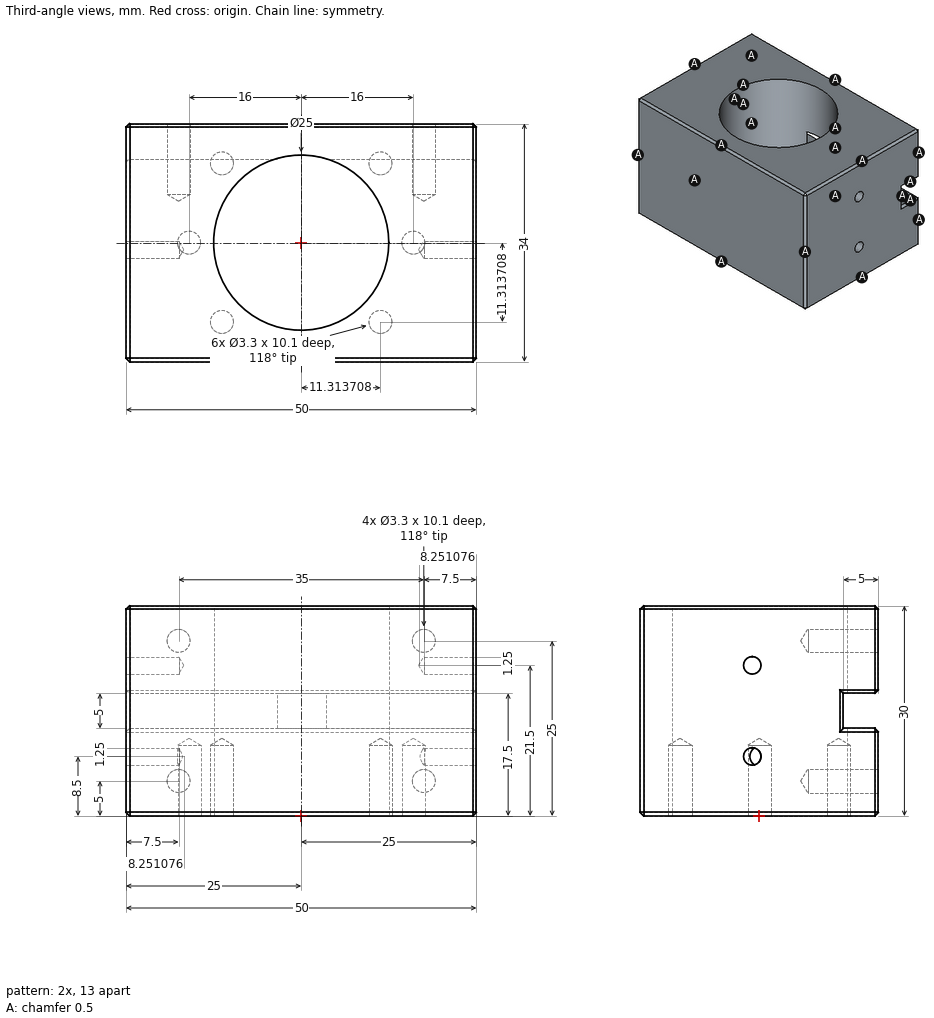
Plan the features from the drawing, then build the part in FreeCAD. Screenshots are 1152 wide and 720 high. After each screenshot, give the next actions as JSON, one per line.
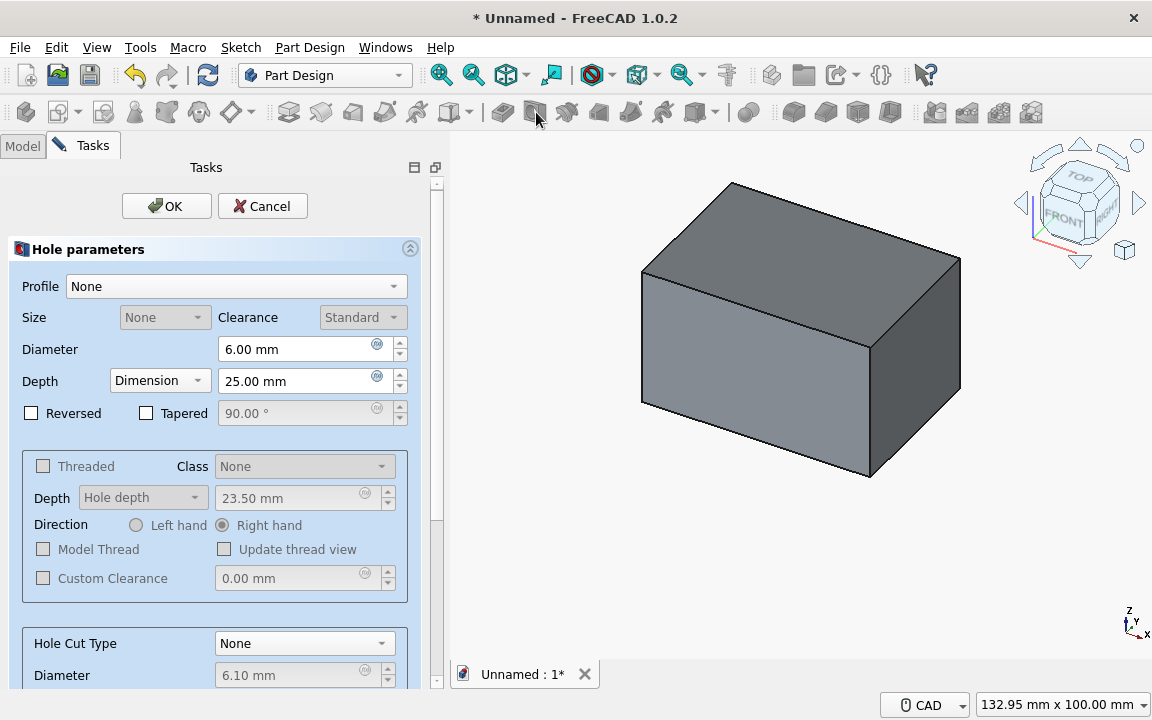
{"action": "triple_click", "coordinate": [305, 349]}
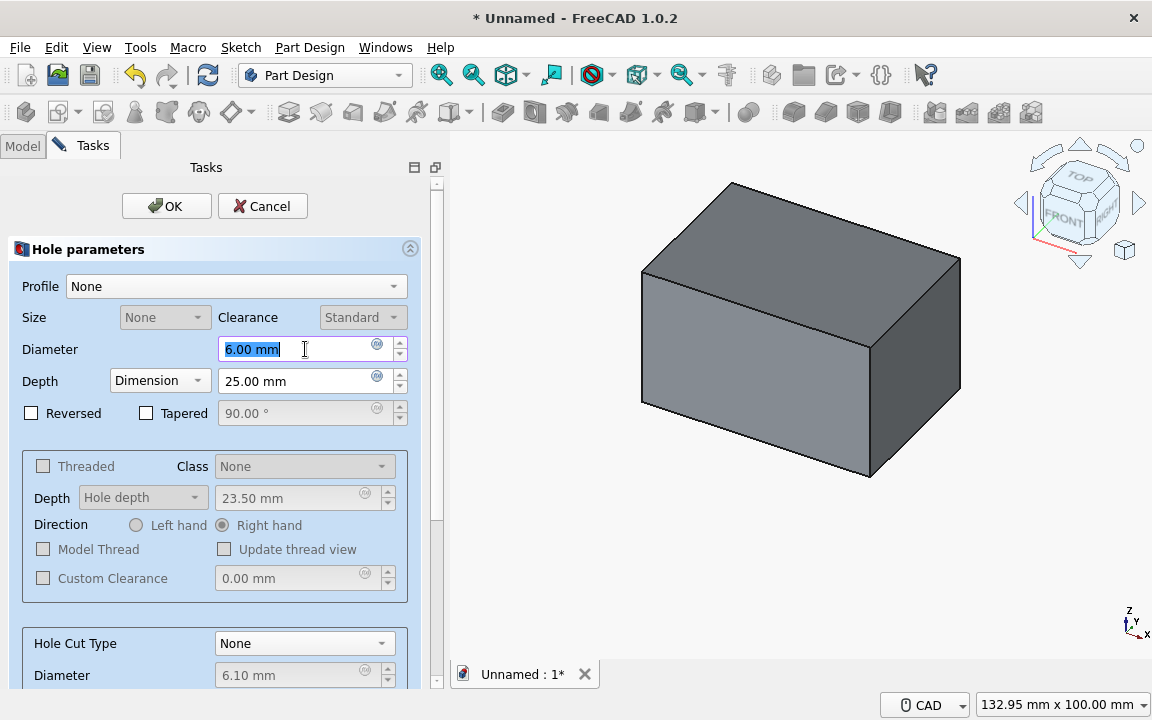
{"action": "type", "text": "3.3"}
{"action": "key", "text": "Tab"}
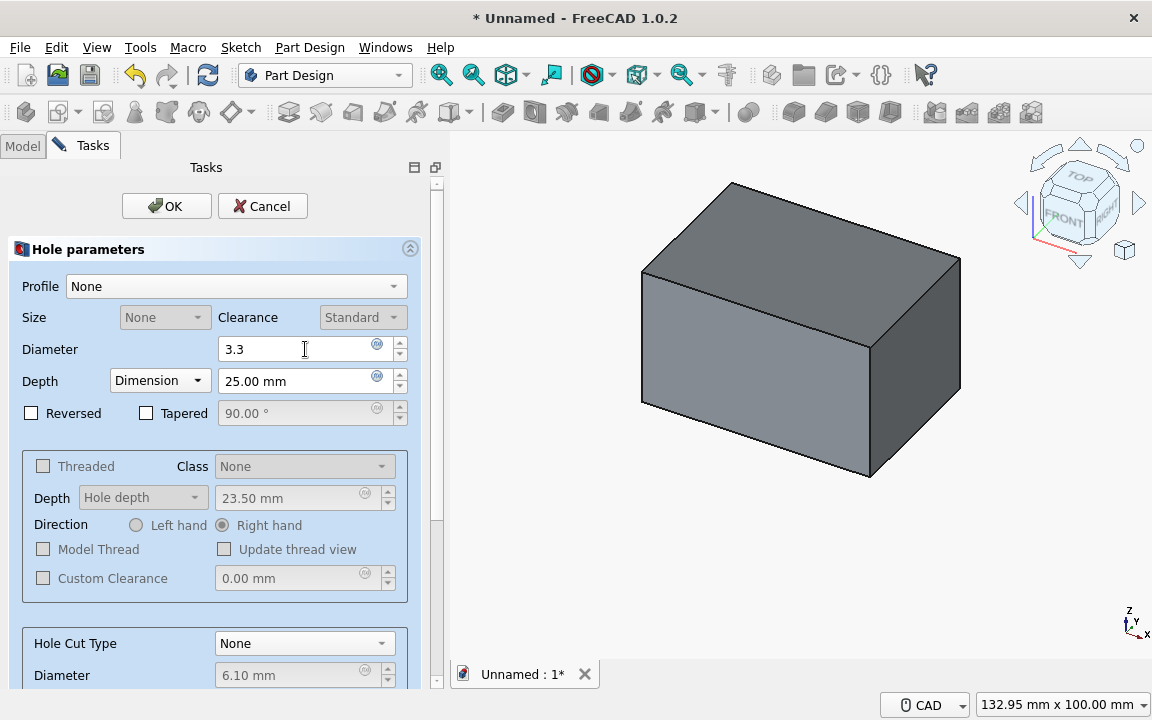
{"action": "triple_click", "coordinate": [305, 381]}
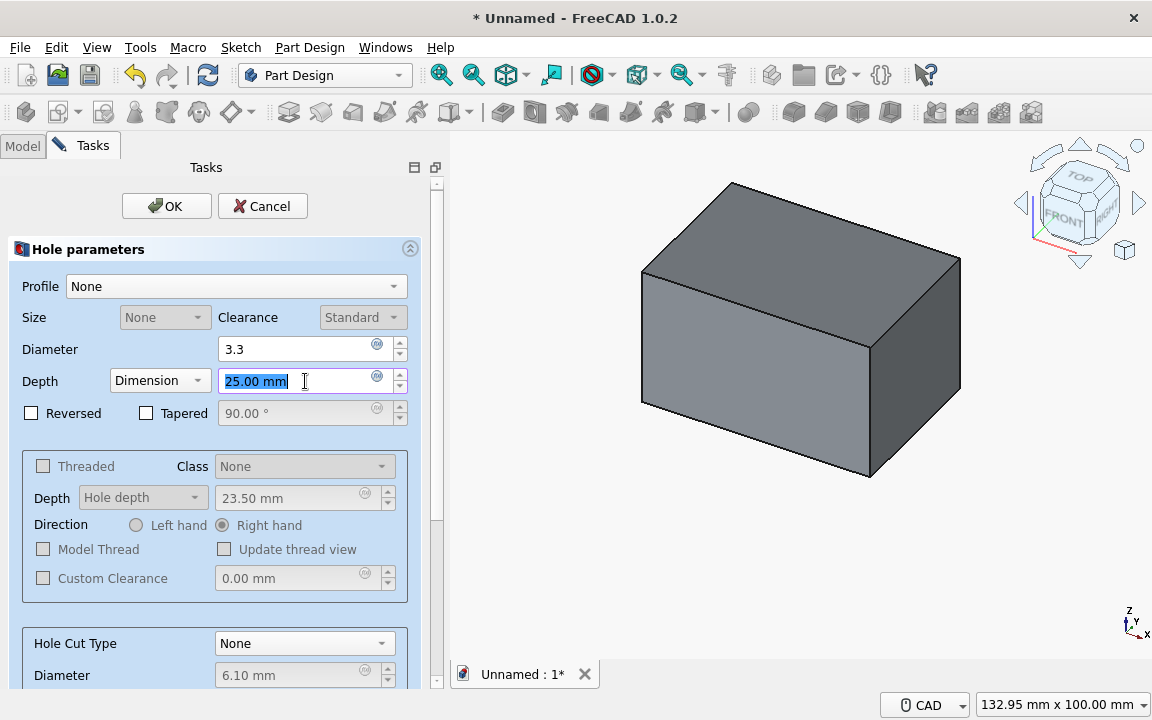
{"action": "type", "text": "10.1"}
{"action": "key", "text": "Tab"}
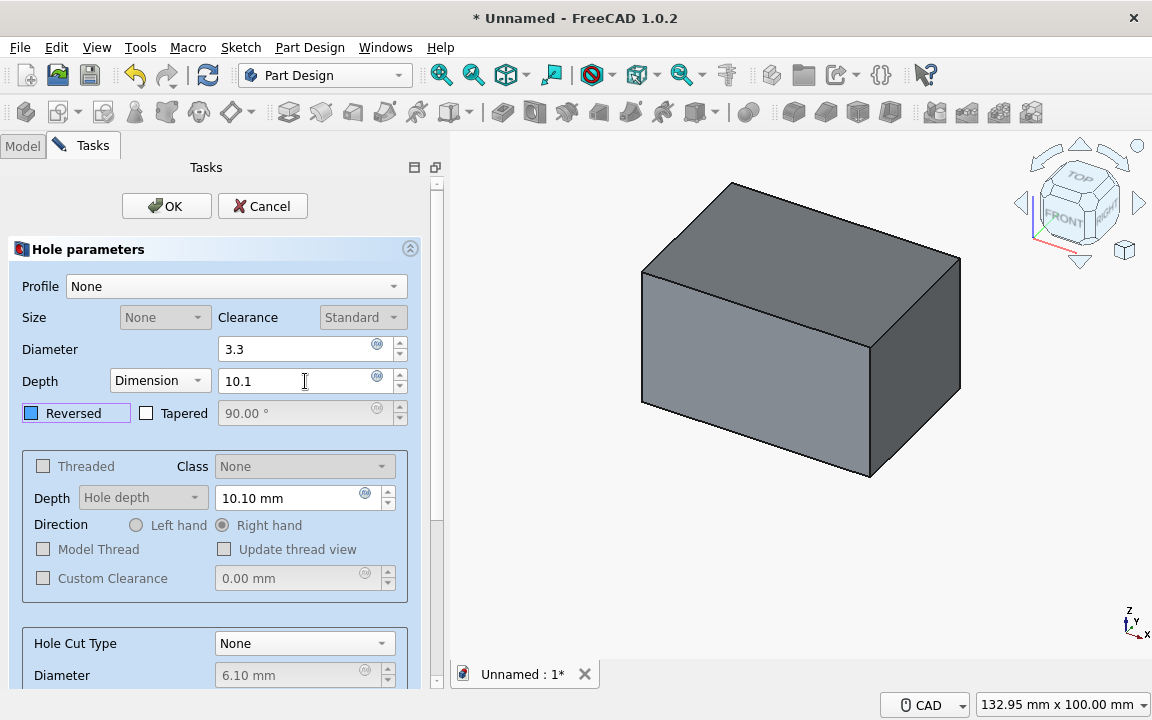
{"action": "left_click", "coordinate": [30, 413]}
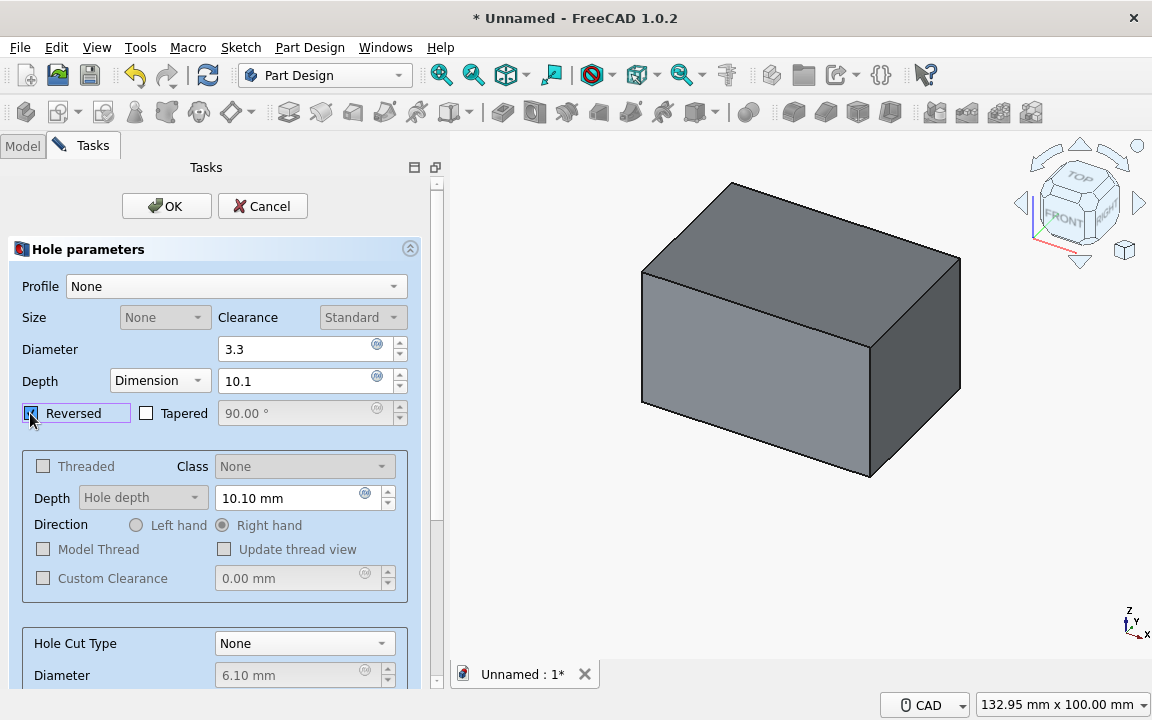
{"action": "left_click", "coordinate": [167, 206]}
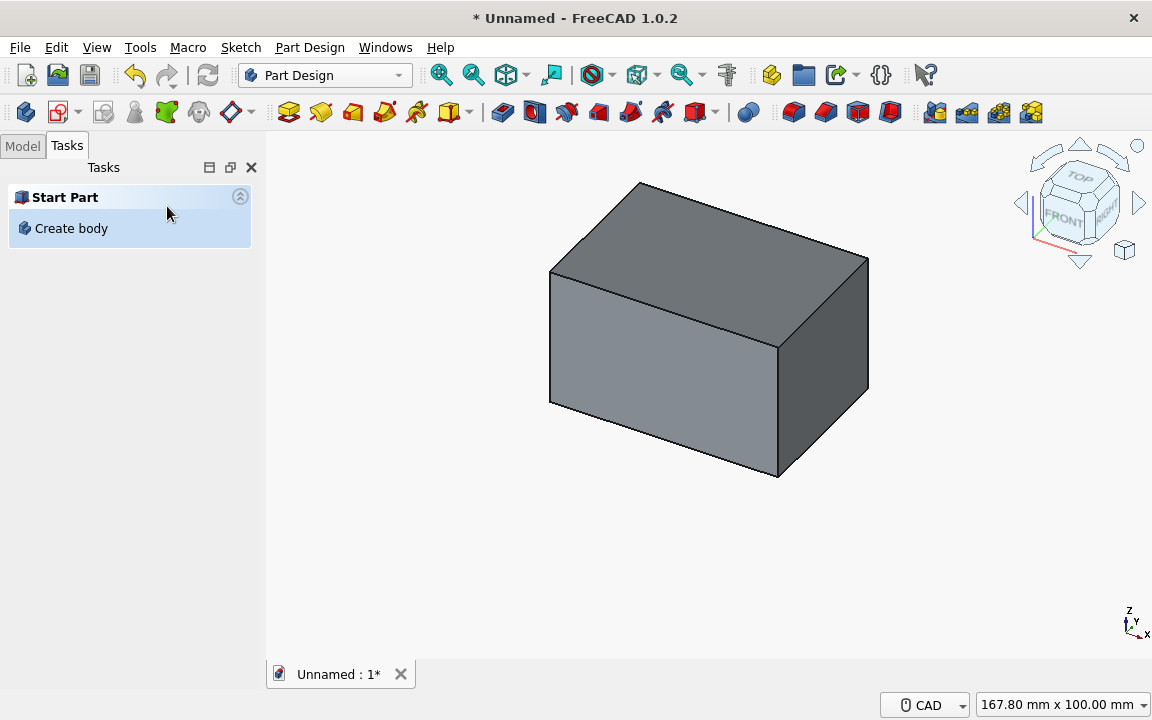
{"action": "left_click", "coordinate": [23, 145]}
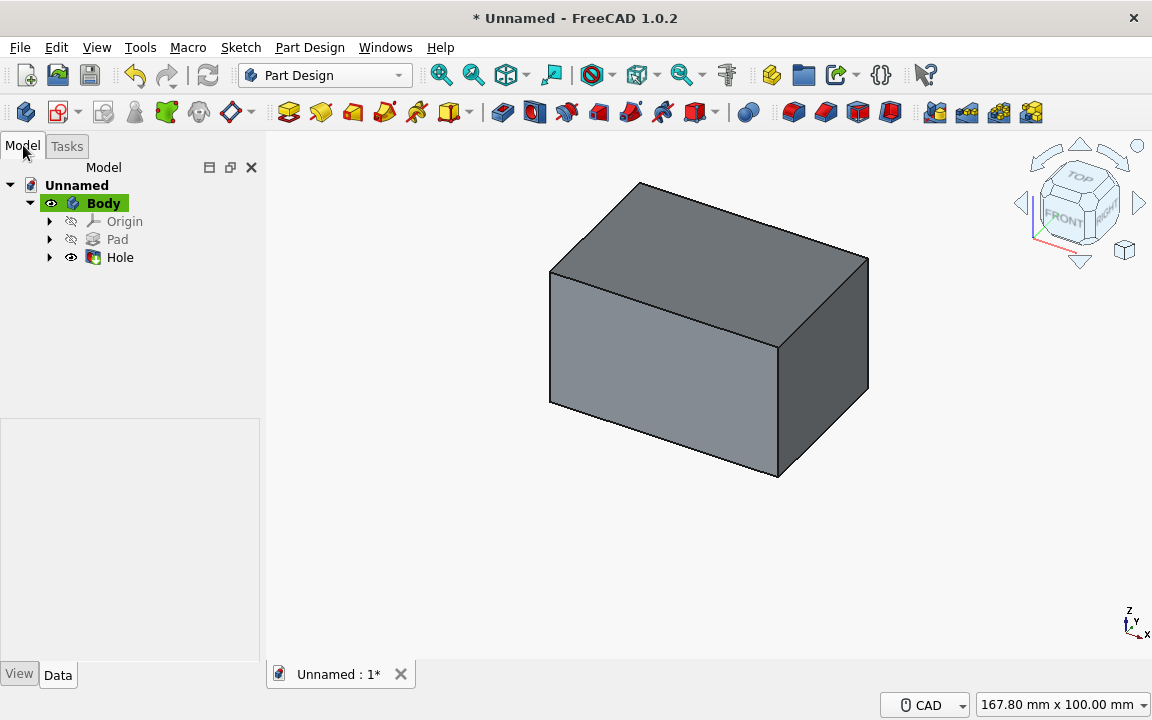
{"action": "left_click", "coordinate": [50, 221]}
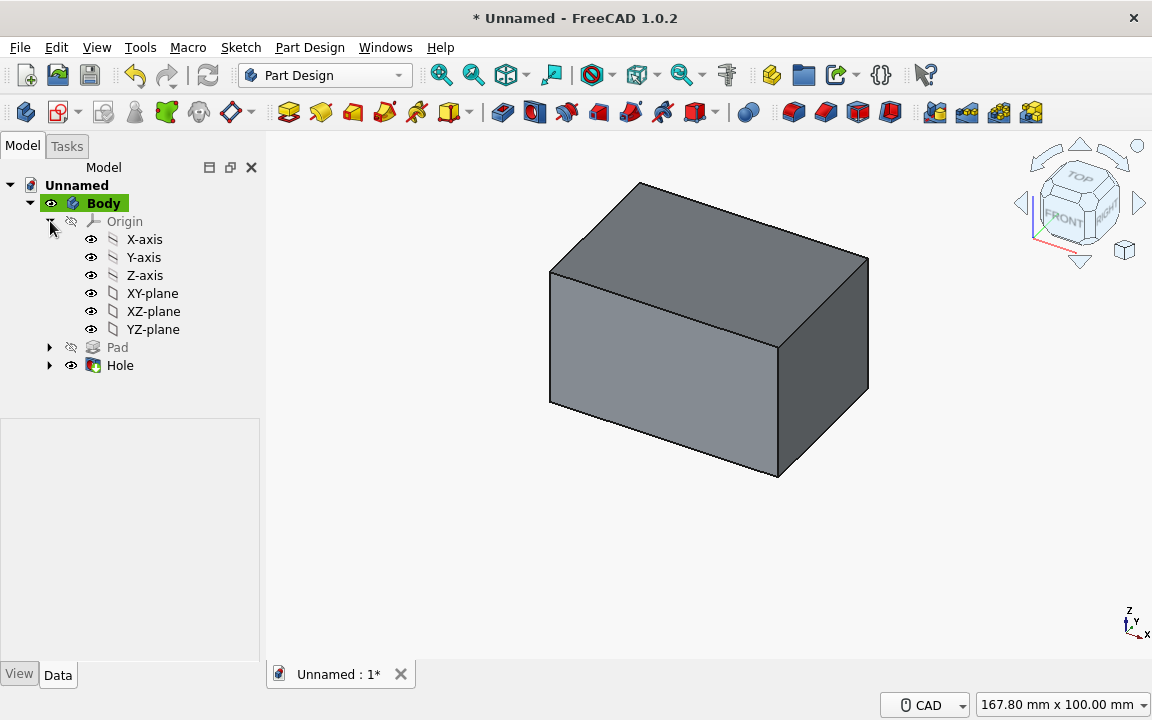
{"action": "left_click", "coordinate": [136, 311]}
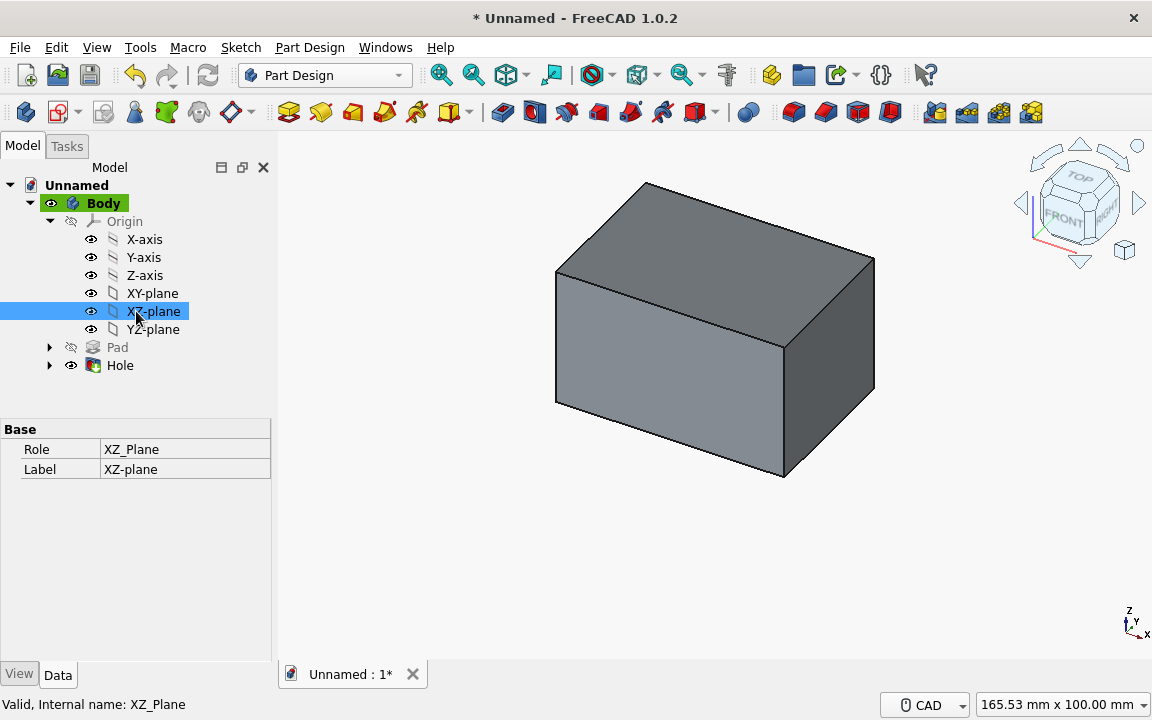
{"action": "left_click", "coordinate": [232, 112]}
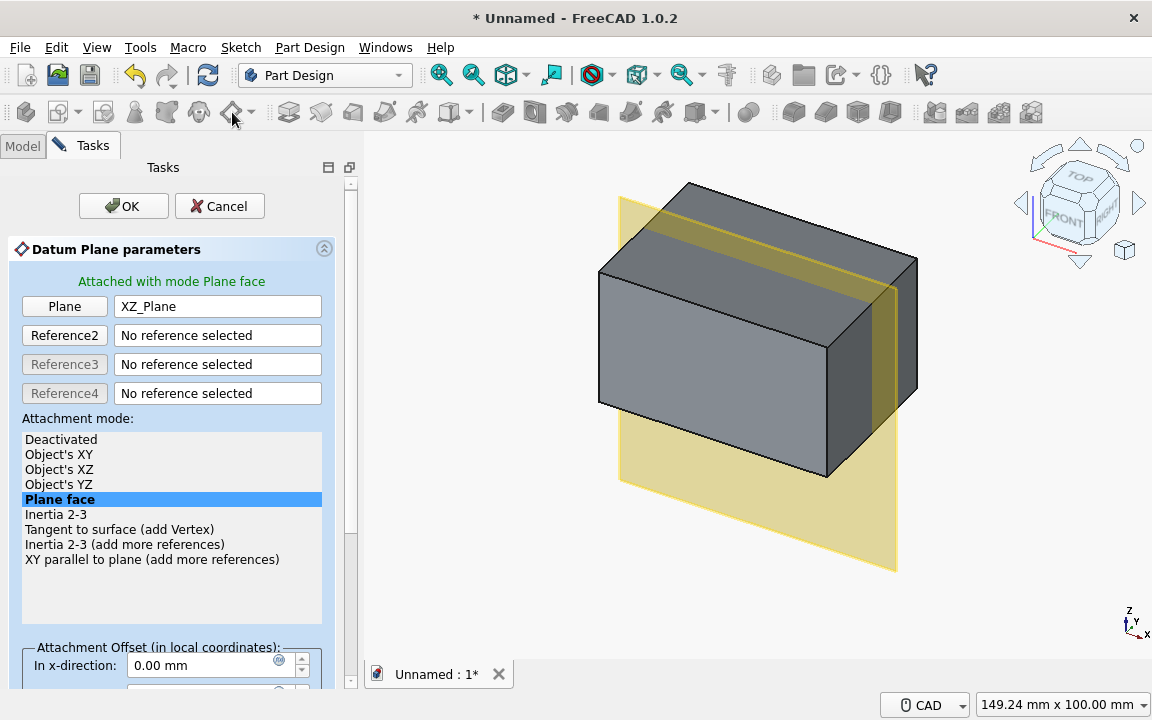
{"action": "scroll", "coordinate": [351, 432], "scroll_direction": "down", "scroll_amount": 2}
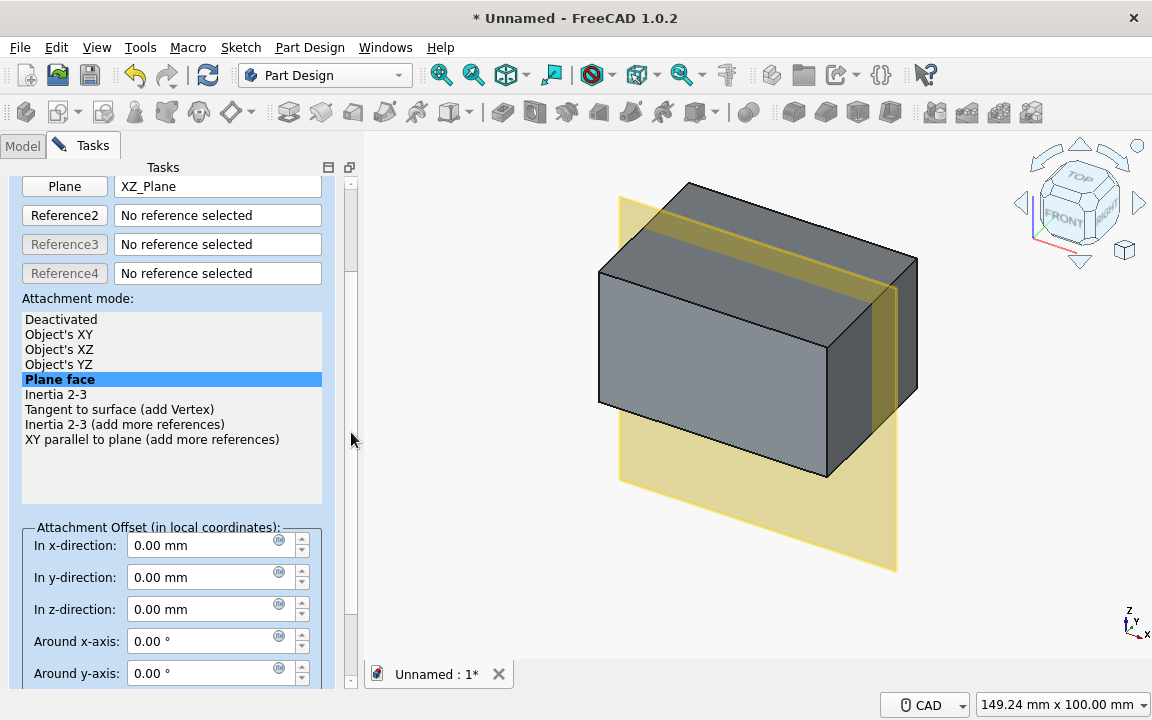
{"action": "triple_click", "coordinate": [210, 609]}